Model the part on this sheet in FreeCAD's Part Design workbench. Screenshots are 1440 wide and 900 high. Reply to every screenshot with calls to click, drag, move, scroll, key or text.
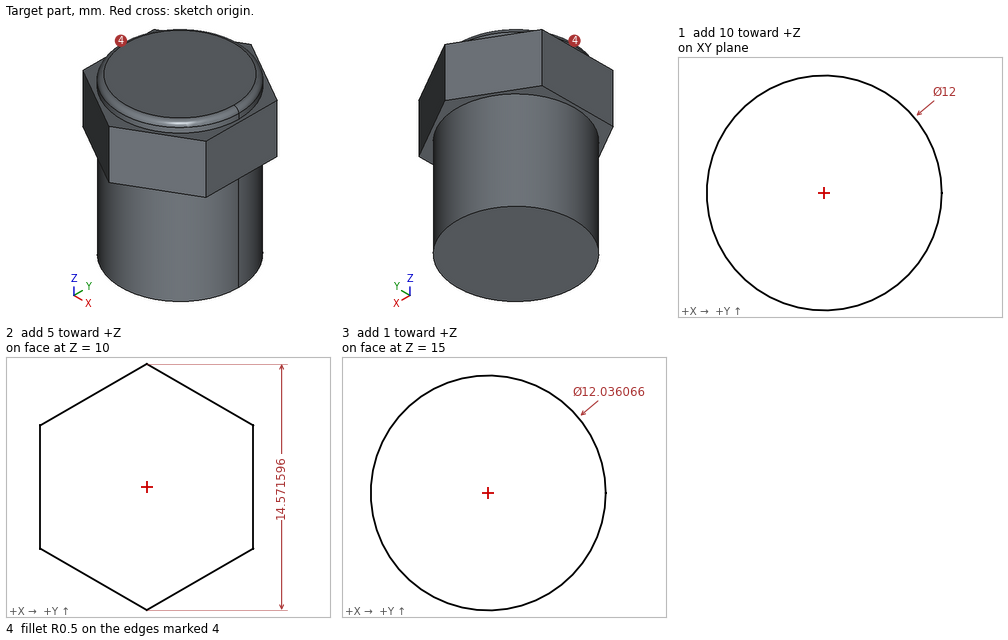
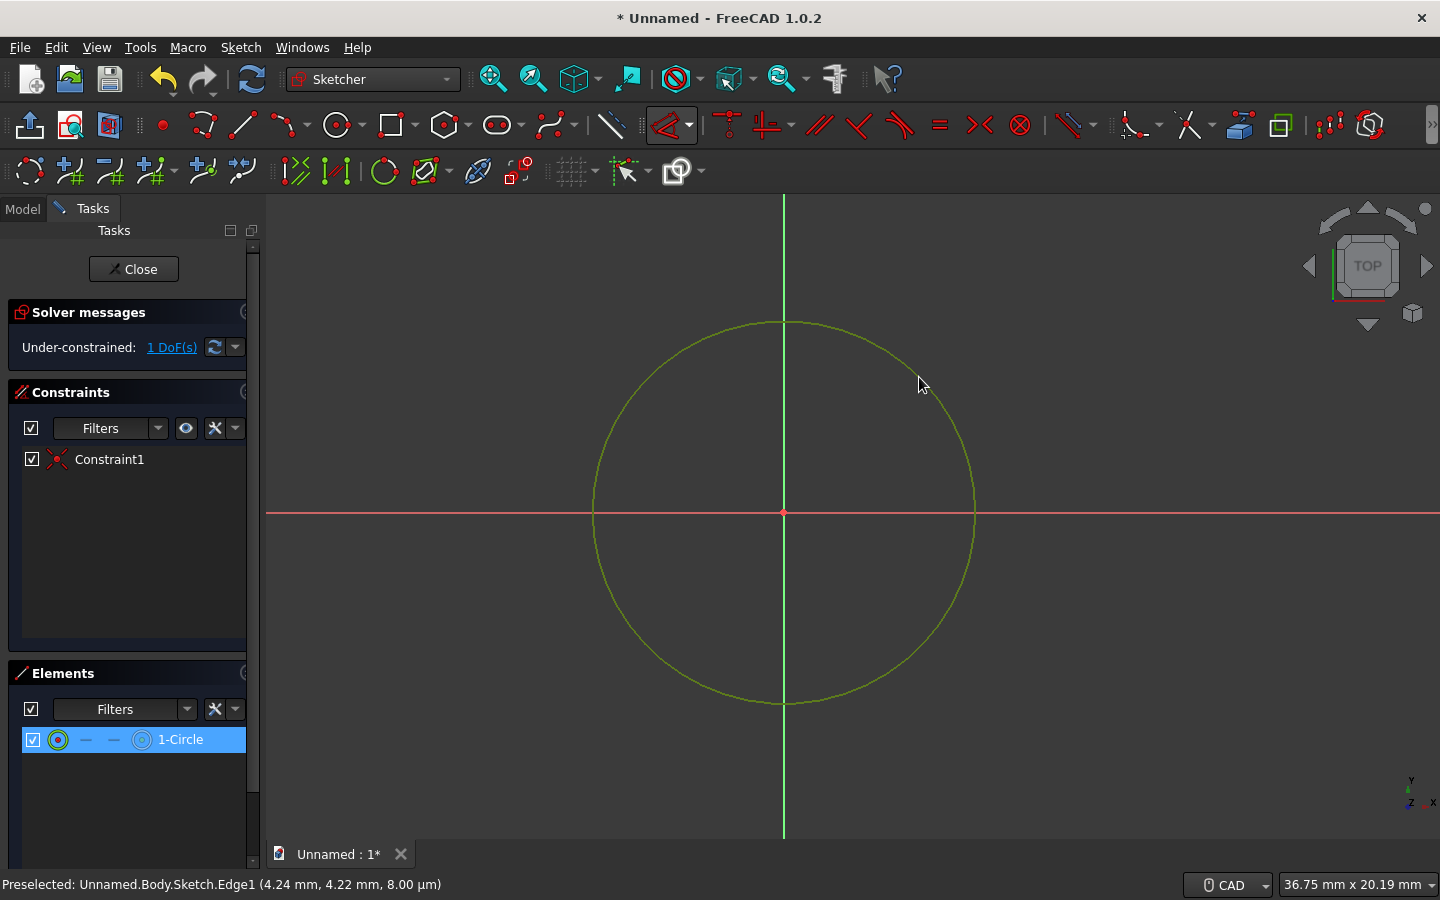
key(k)
key(o)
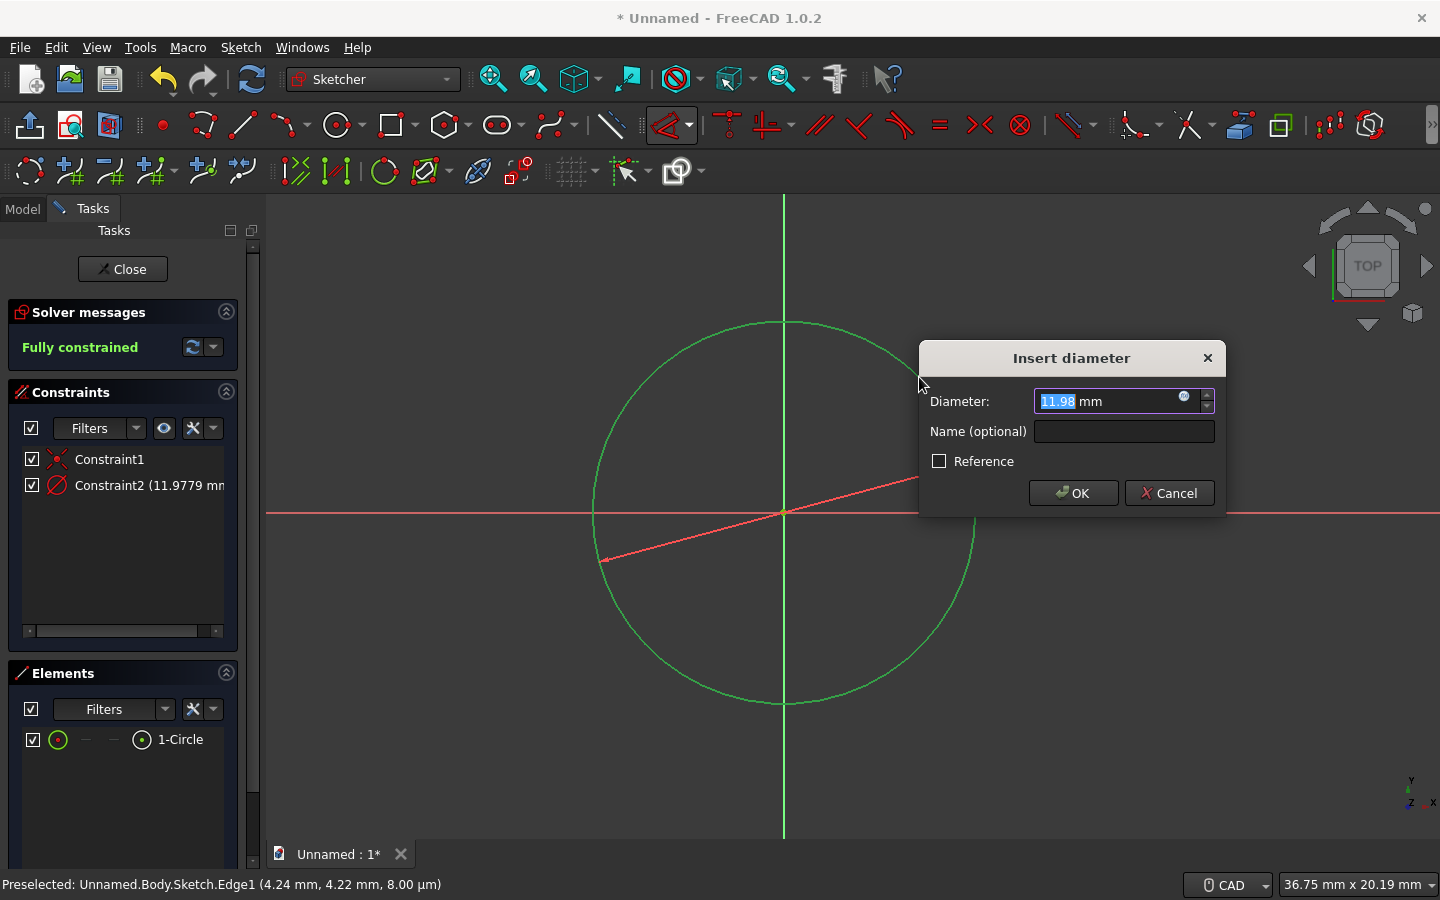
text(12)
key(Return)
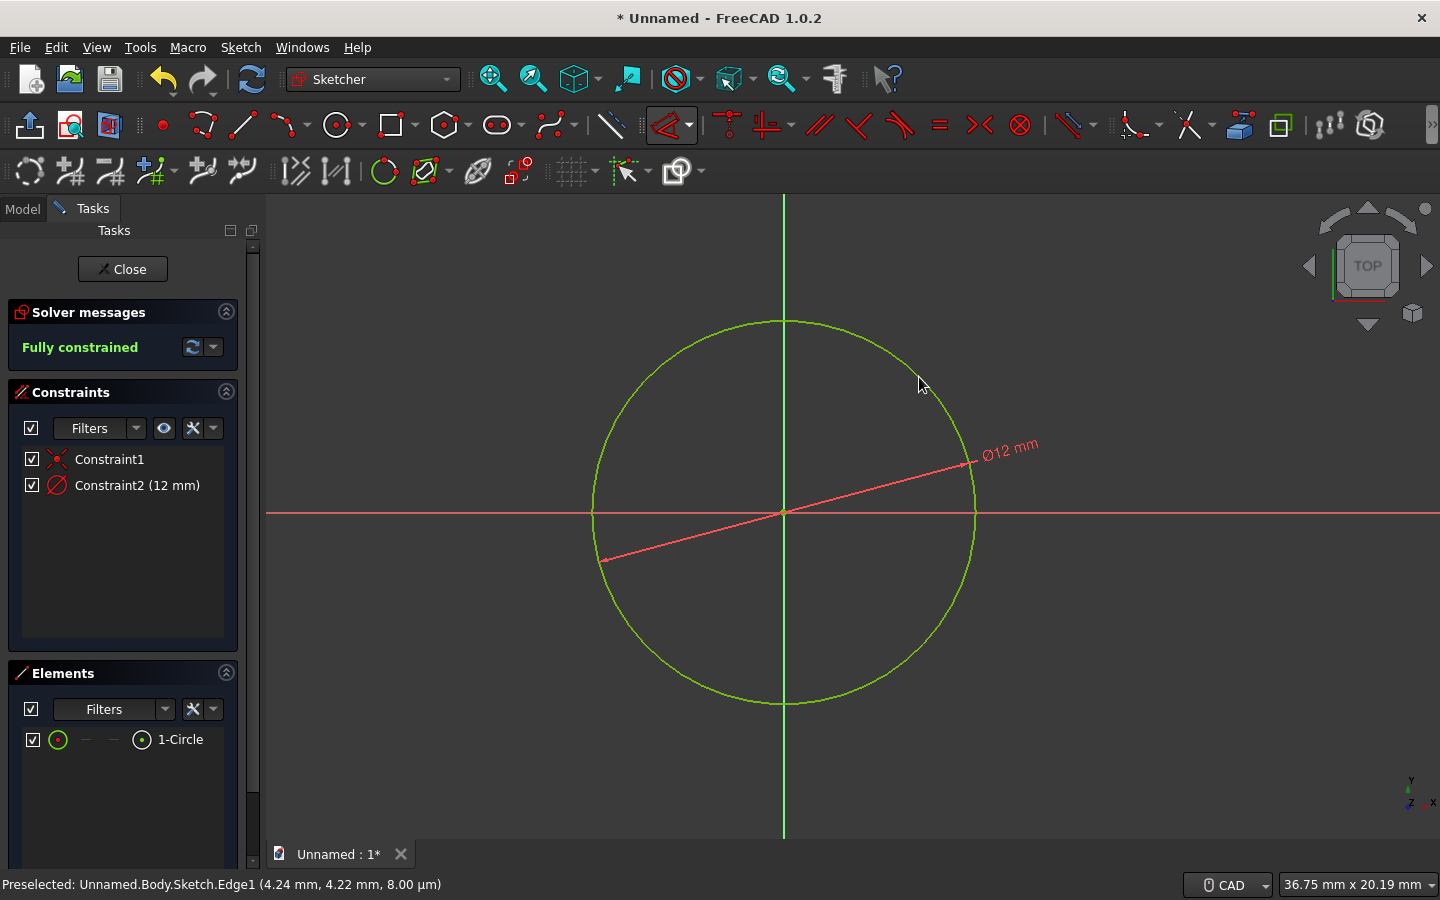
click(123, 269)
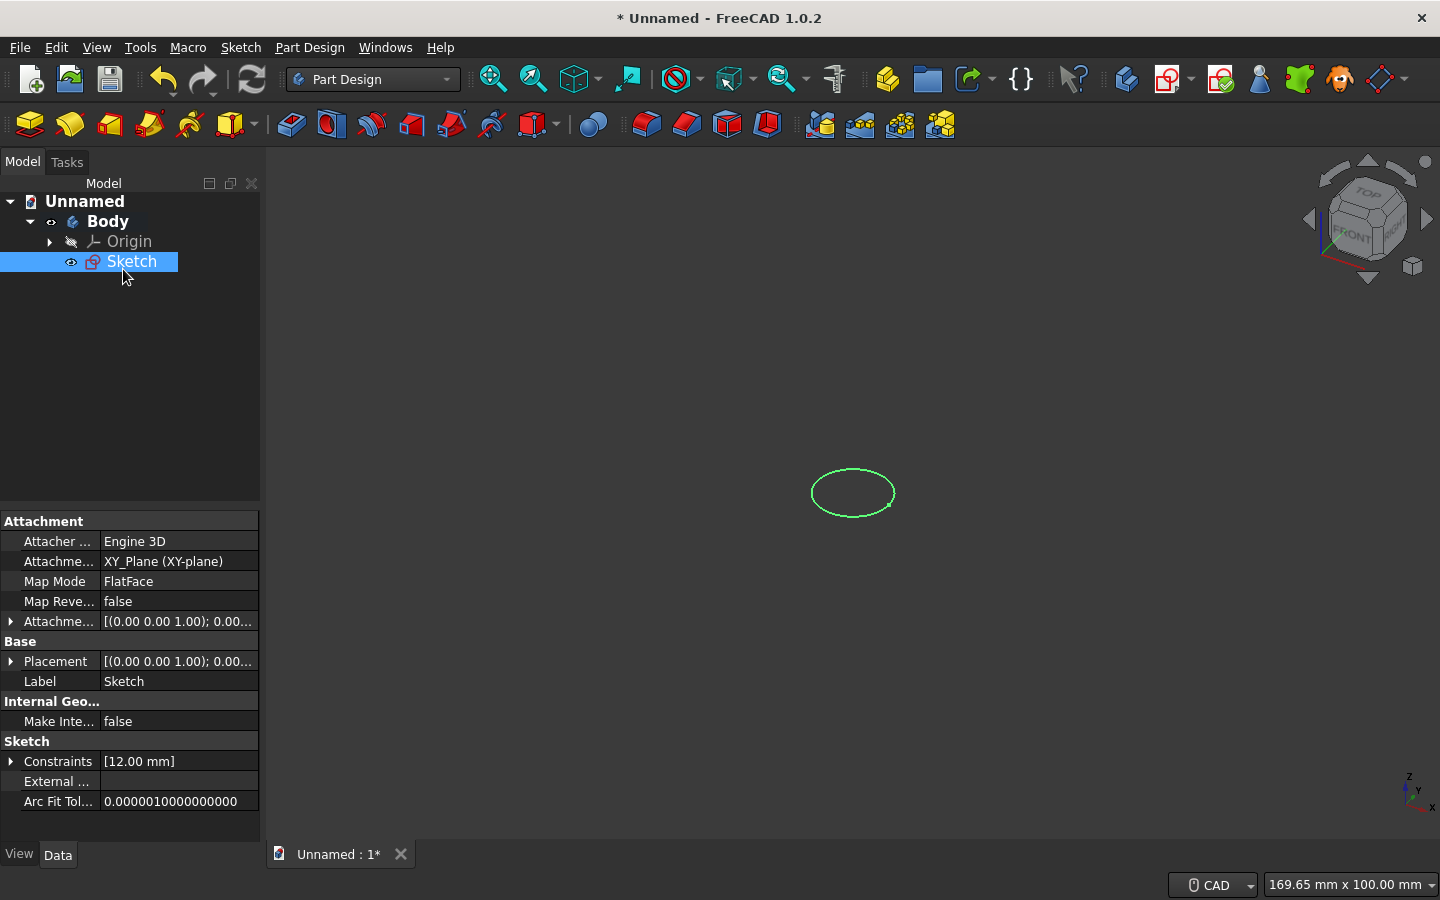
click(30, 124)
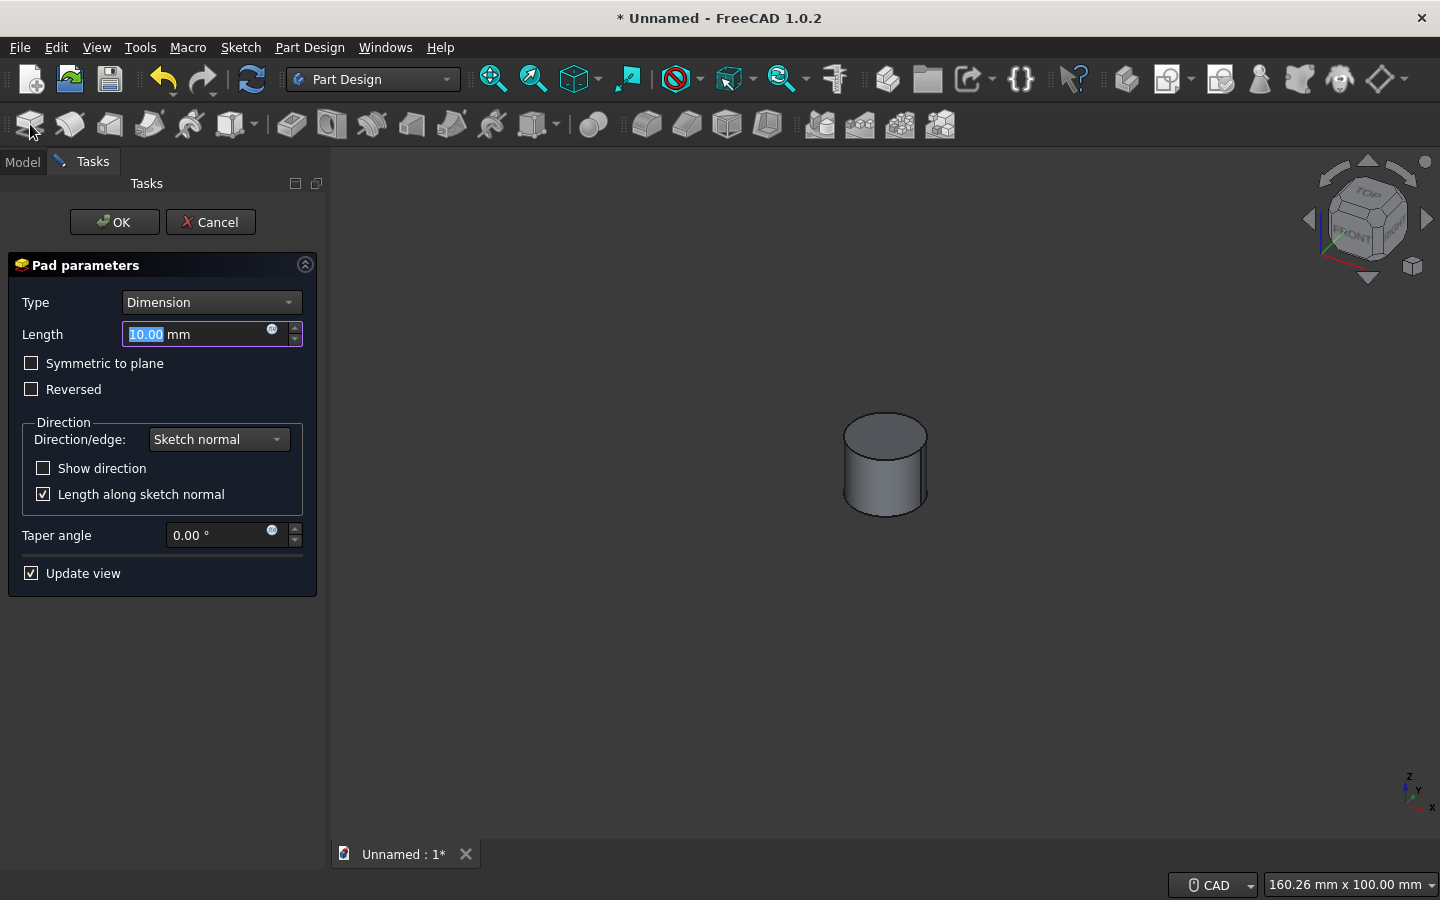
text(10)
key(Tab)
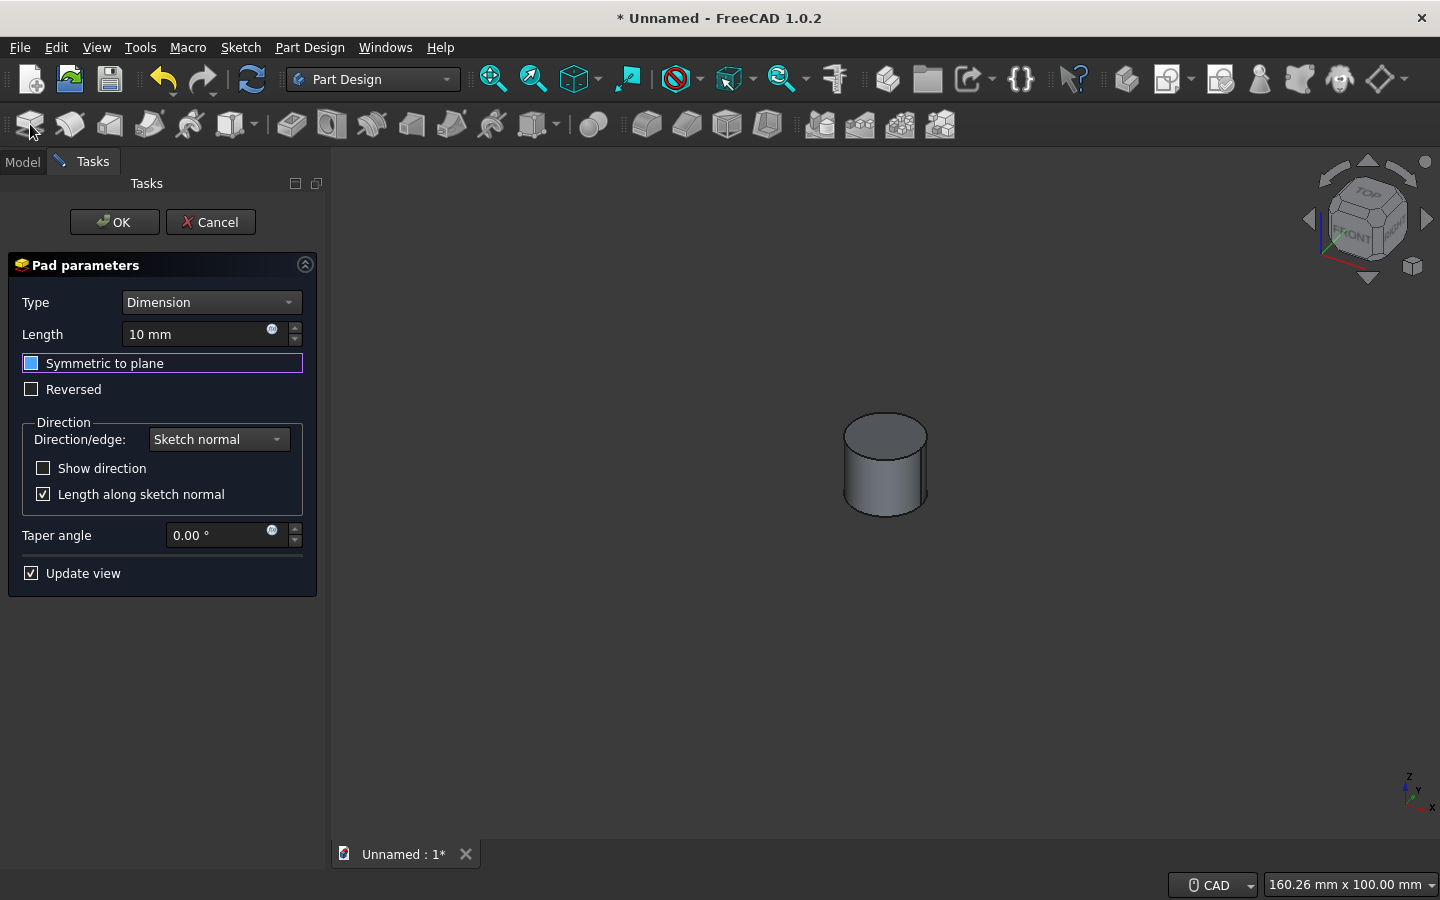
click(115, 222)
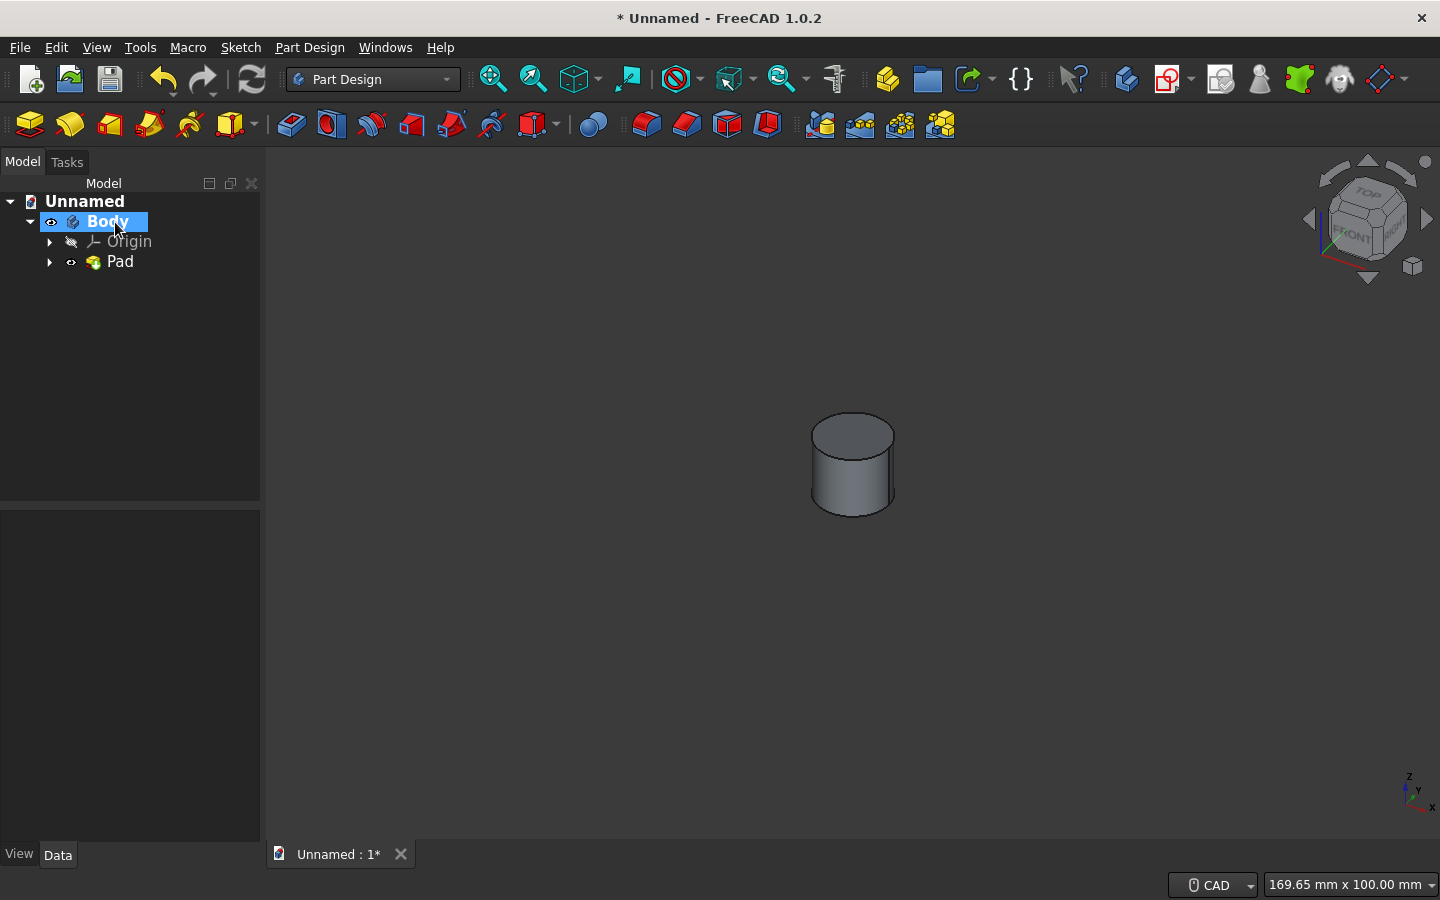
click(494, 80)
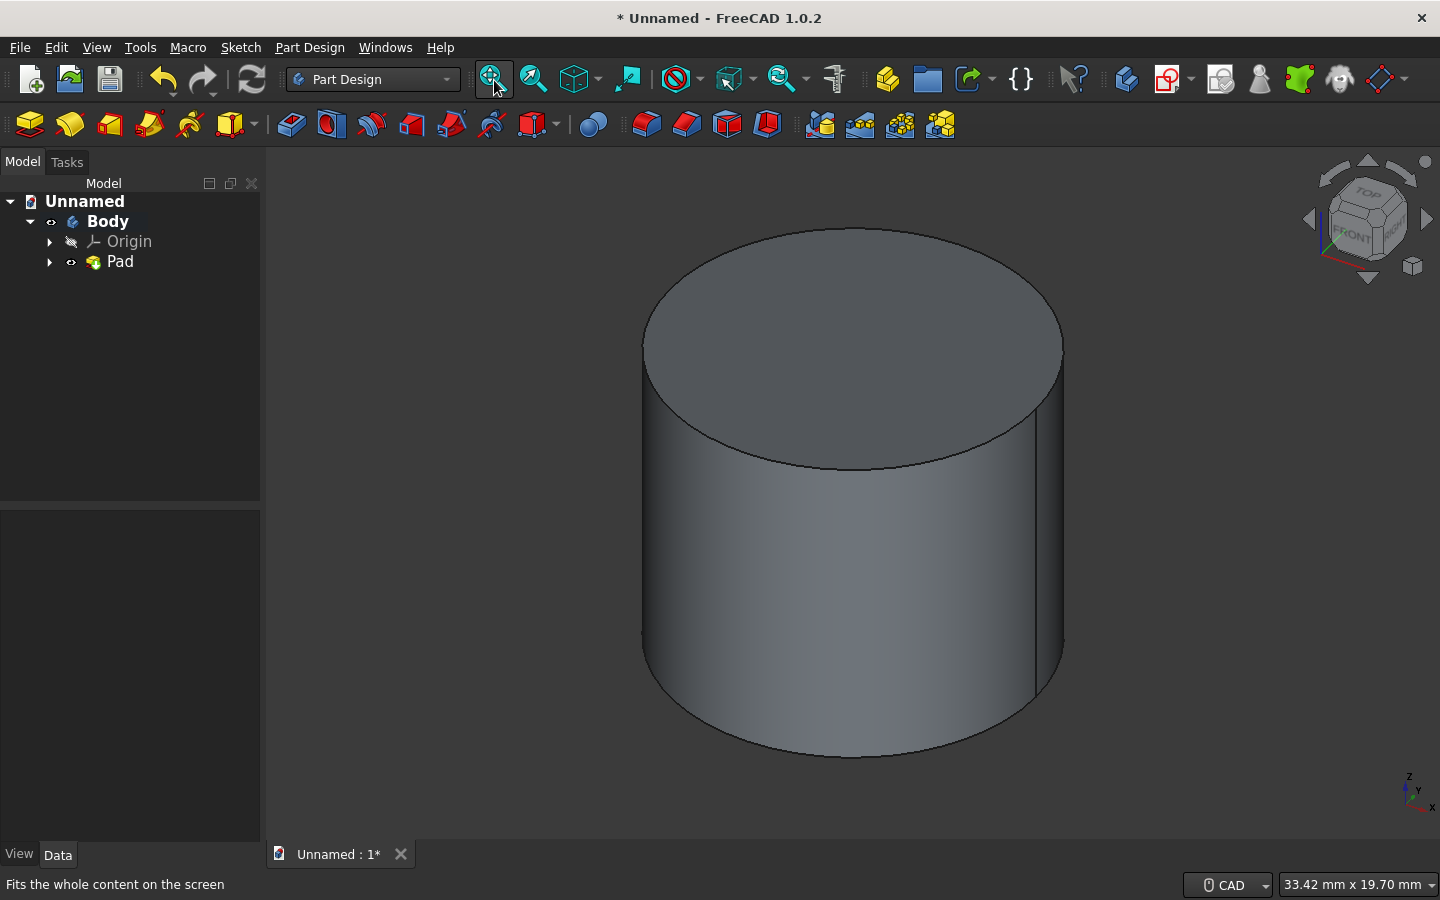
click(853, 348)